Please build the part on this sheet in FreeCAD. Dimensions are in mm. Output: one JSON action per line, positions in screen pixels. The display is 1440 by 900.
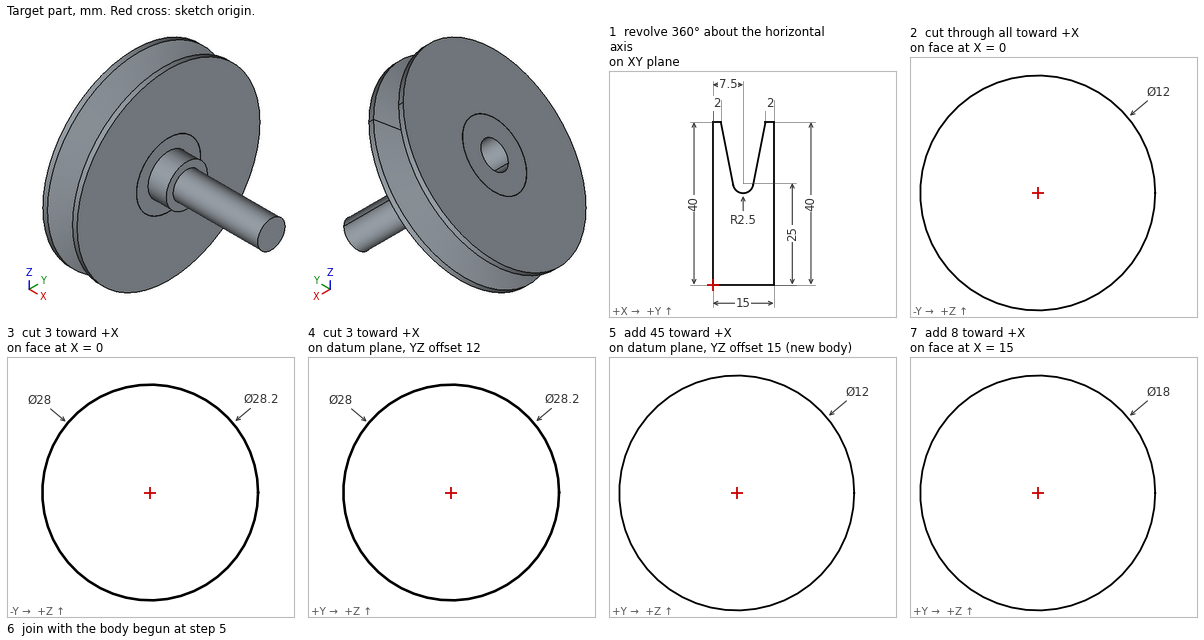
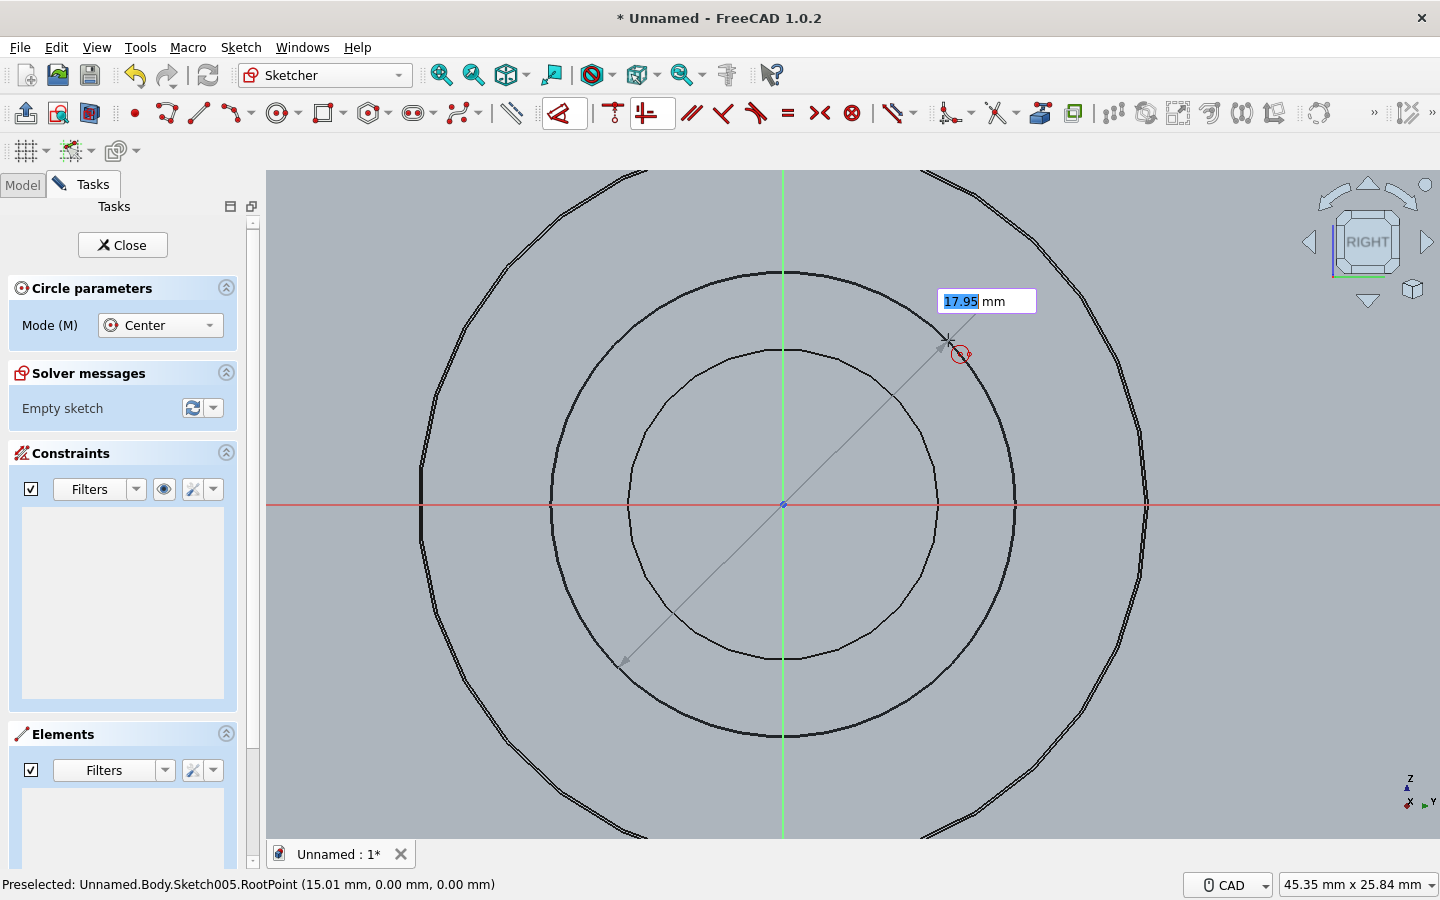
{"action": "type", "text": "18"}
{"action": "key", "text": "Return"}
{"action": "key", "text": "Escape"}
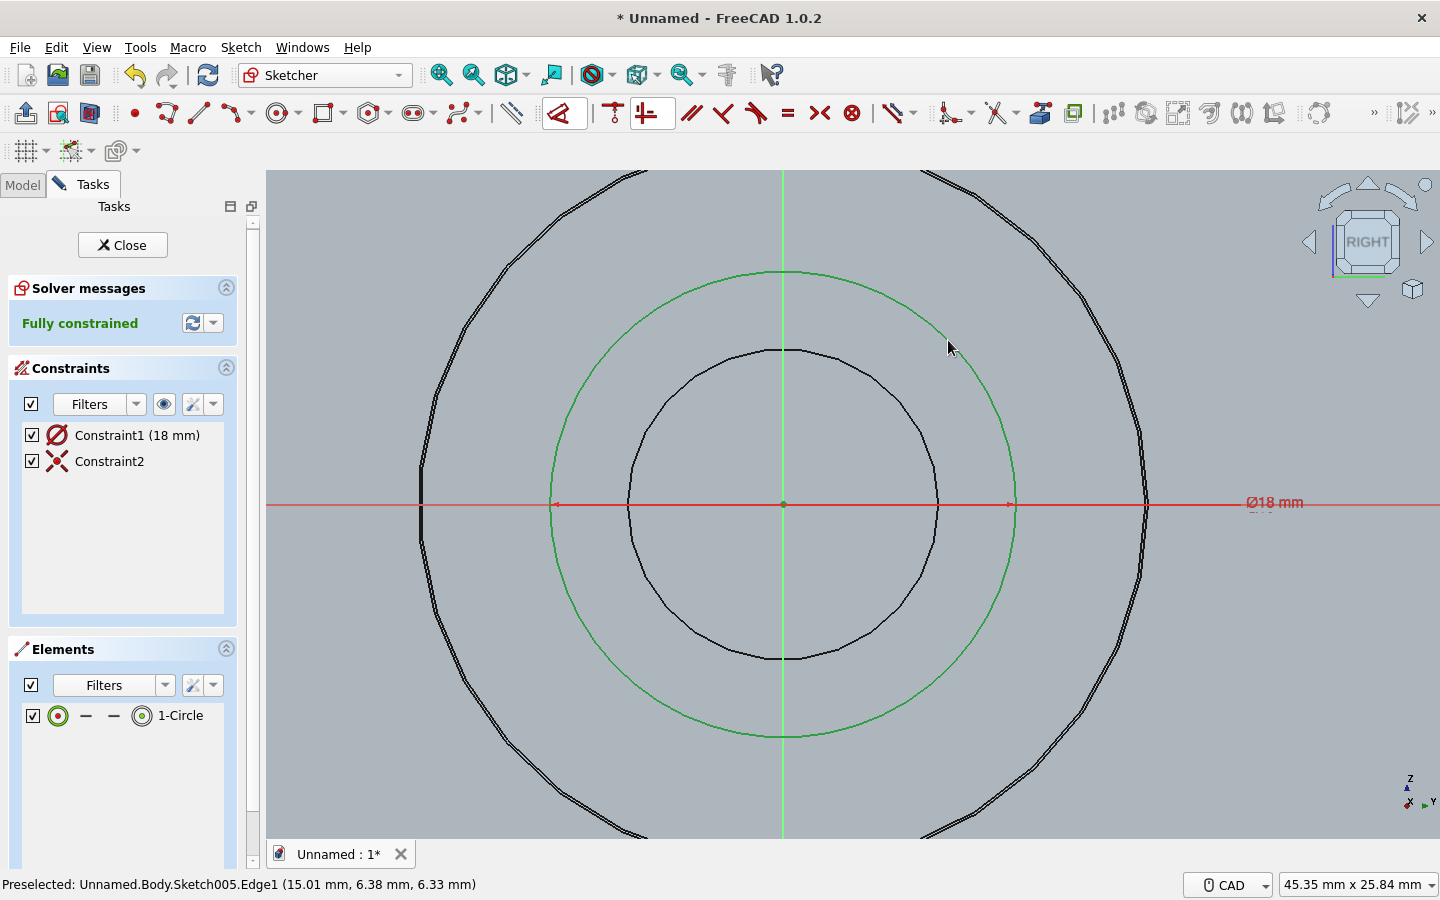
{"action": "left_click", "coordinate": [123, 245]}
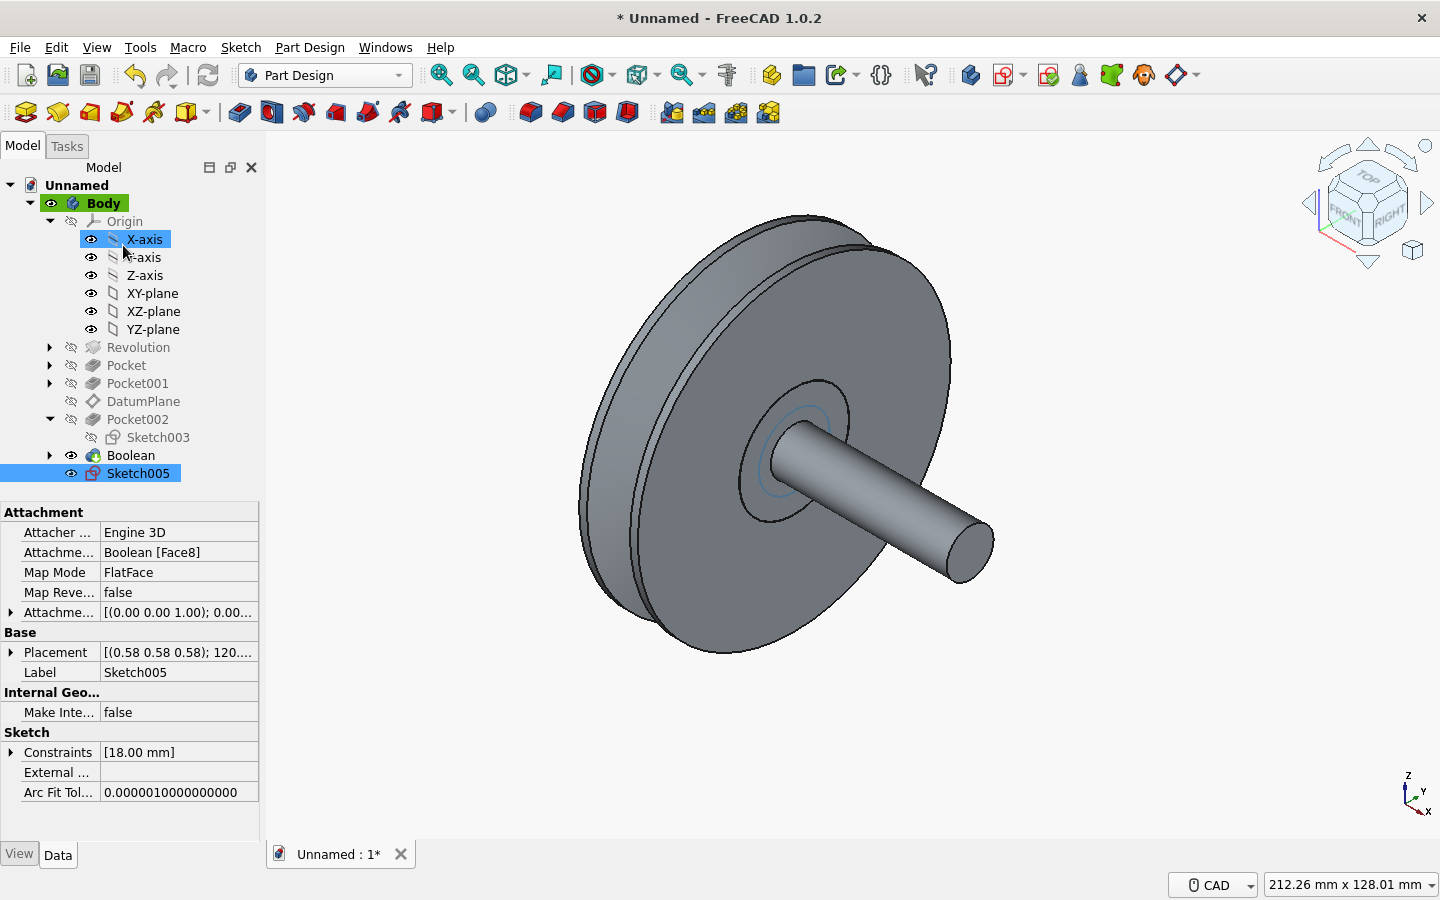
{"action": "left_click", "coordinate": [26, 112]}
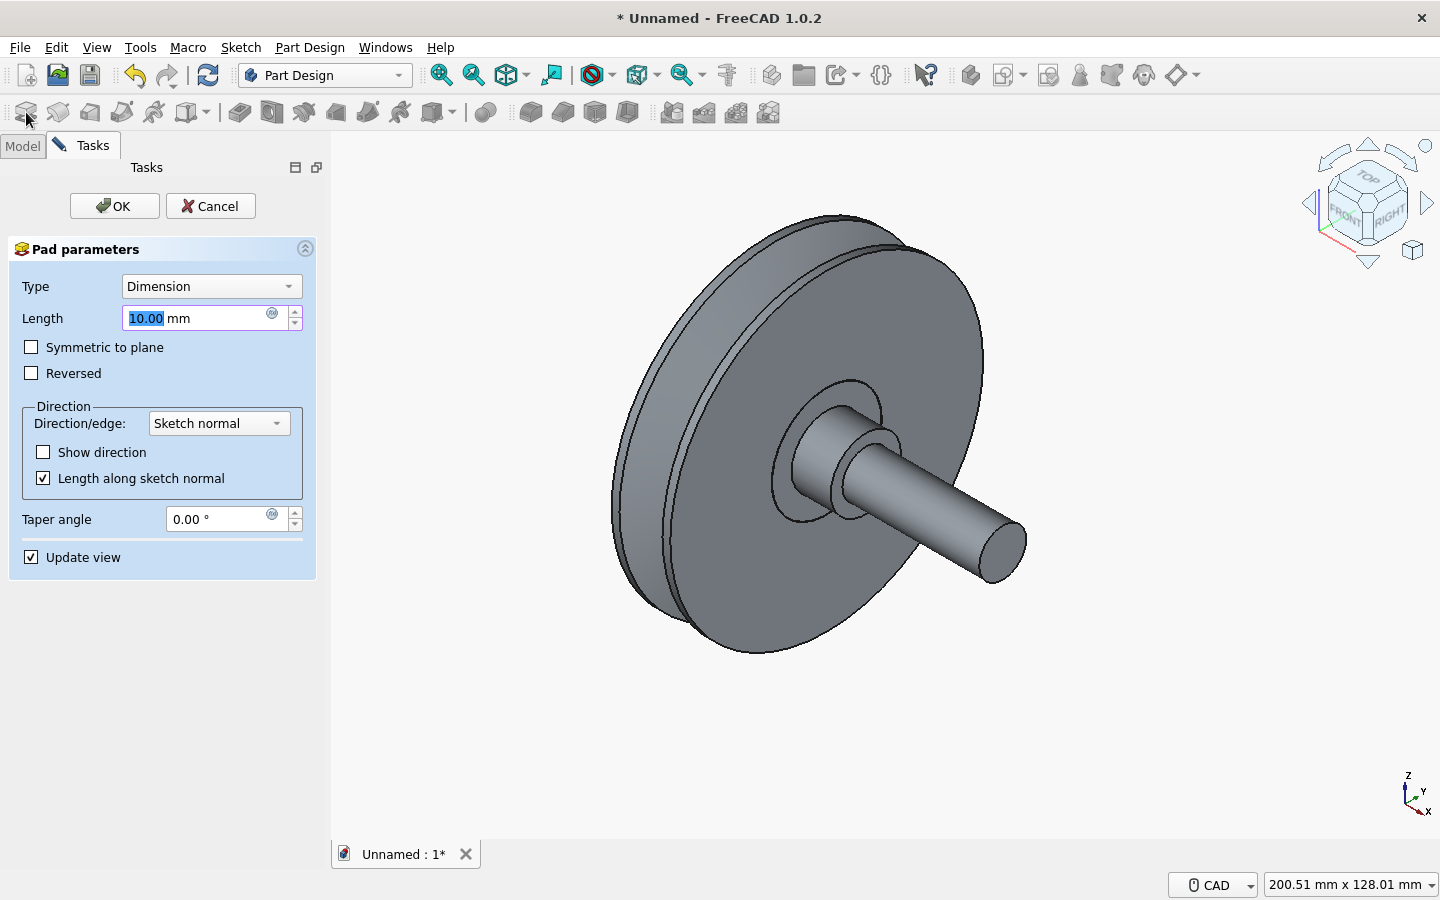
{"action": "type", "text": "8"}
{"action": "key", "text": "Tab"}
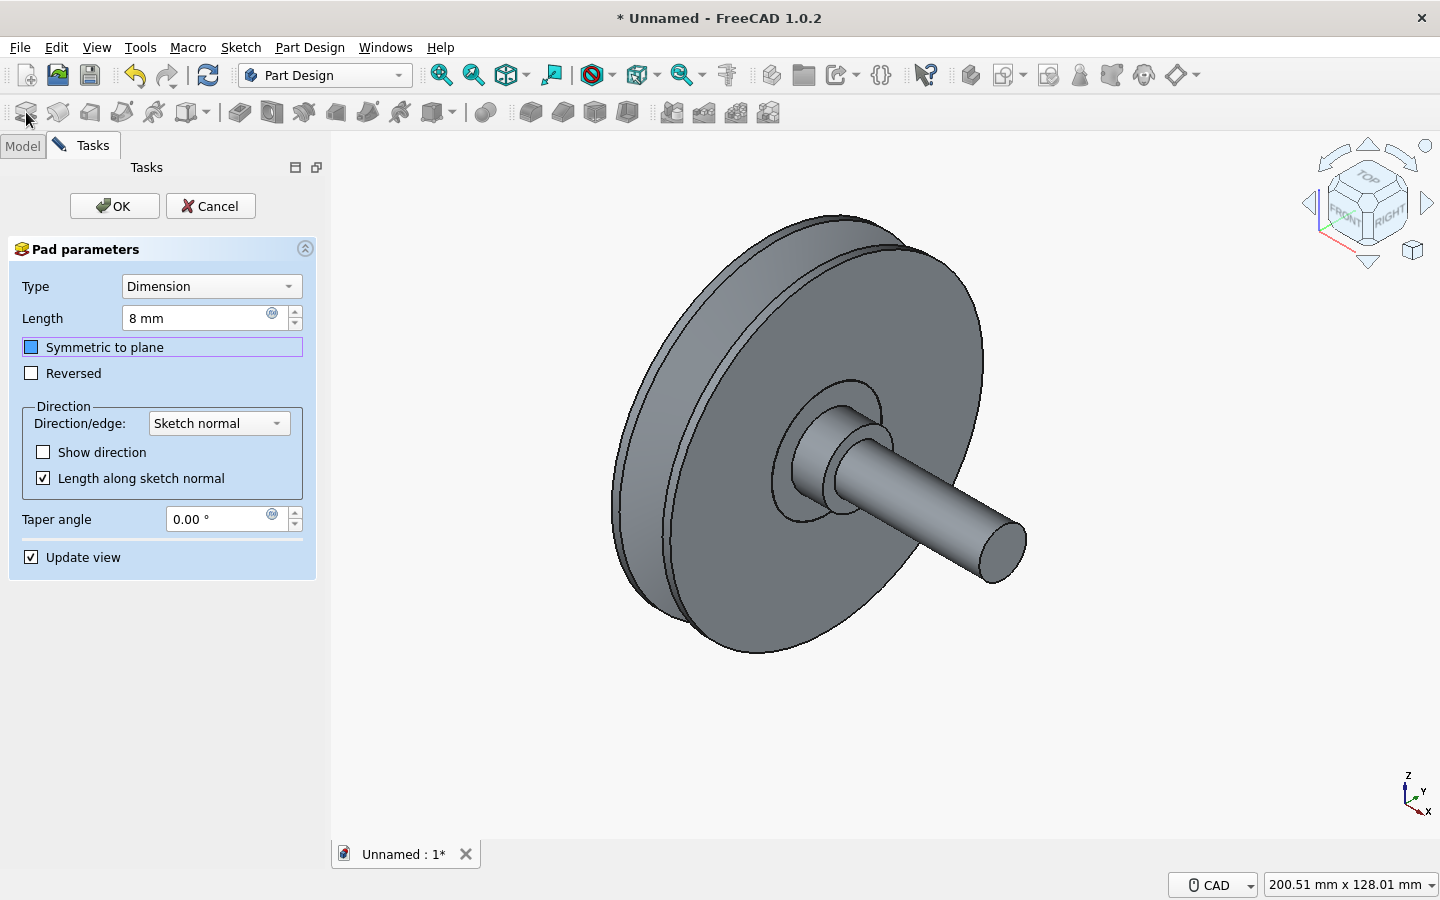
{"action": "left_click", "coordinate": [115, 206]}